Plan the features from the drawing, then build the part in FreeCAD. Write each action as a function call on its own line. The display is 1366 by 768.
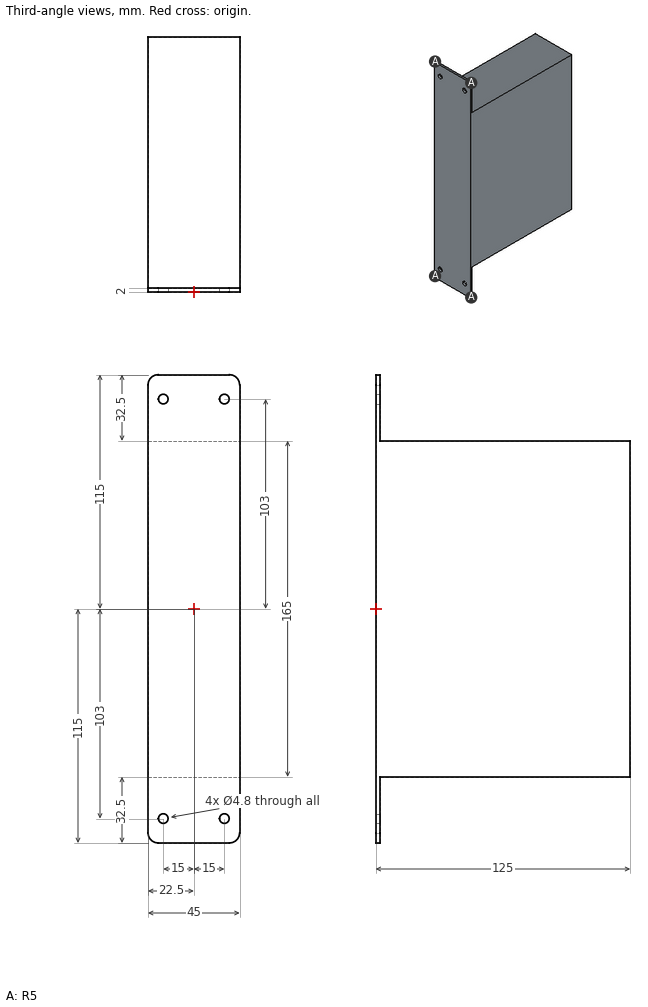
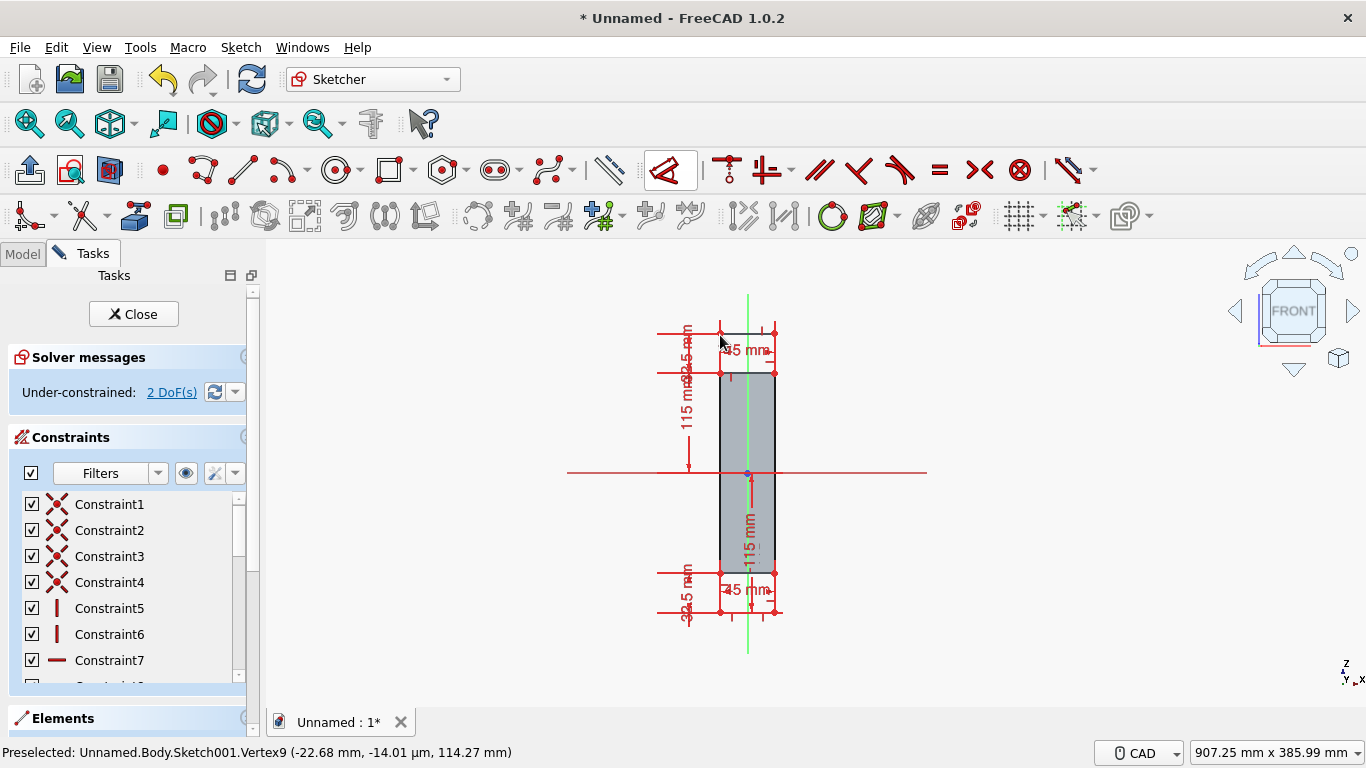
scroll(720, 573, up, 2)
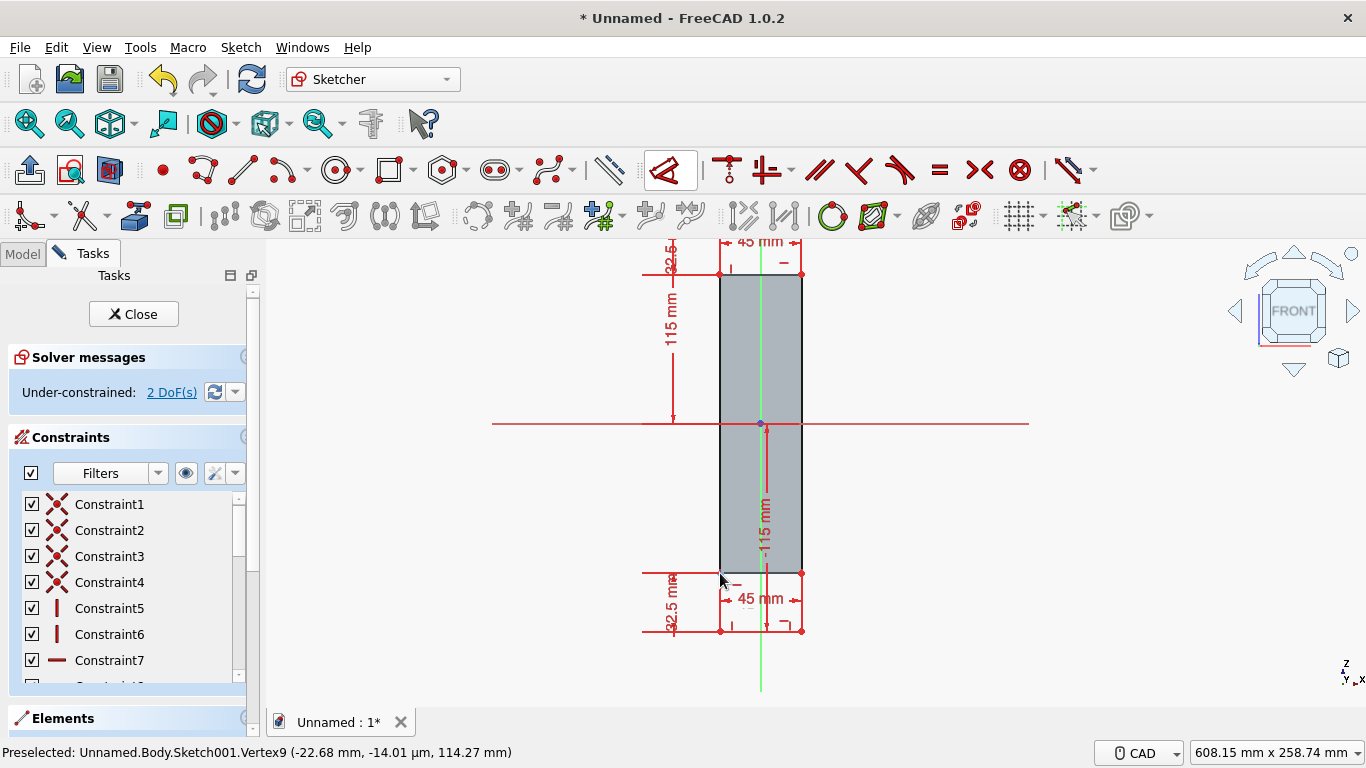
click(720, 573)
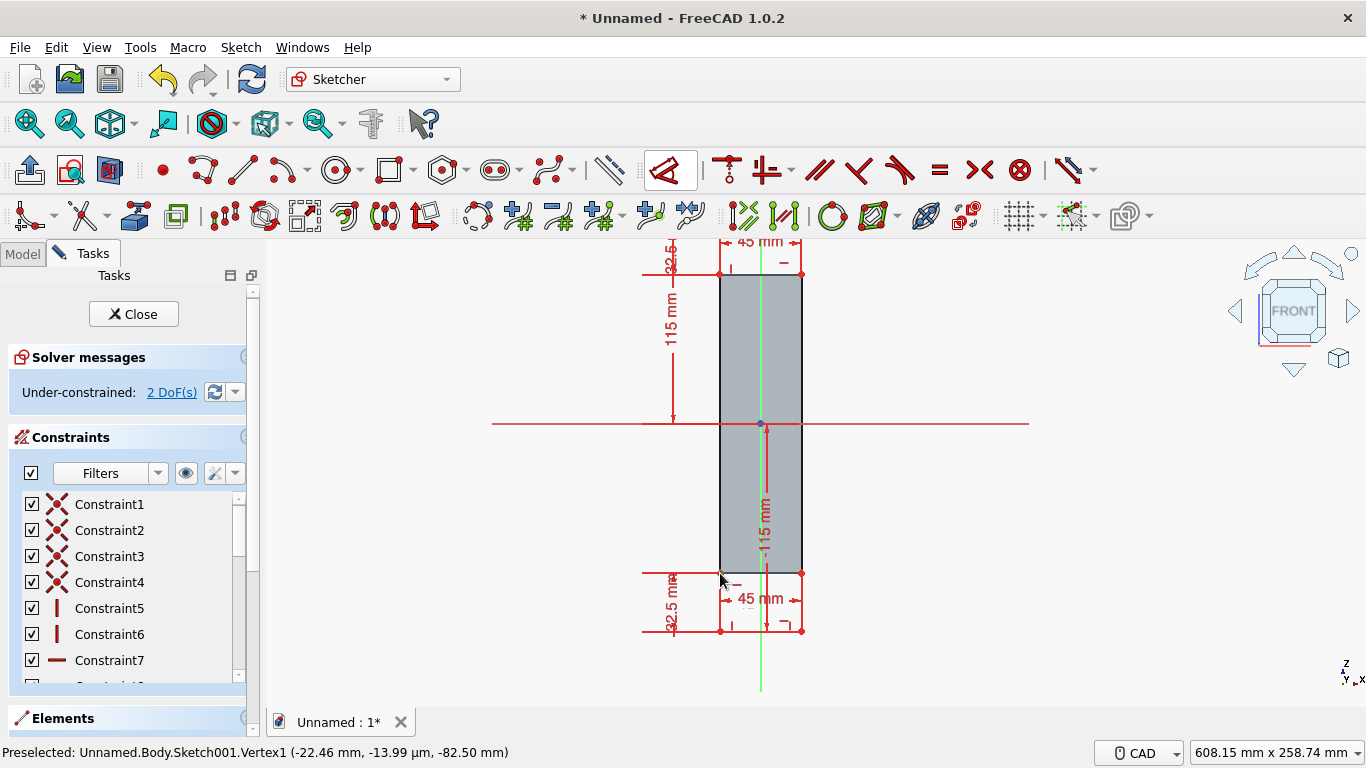
key(l)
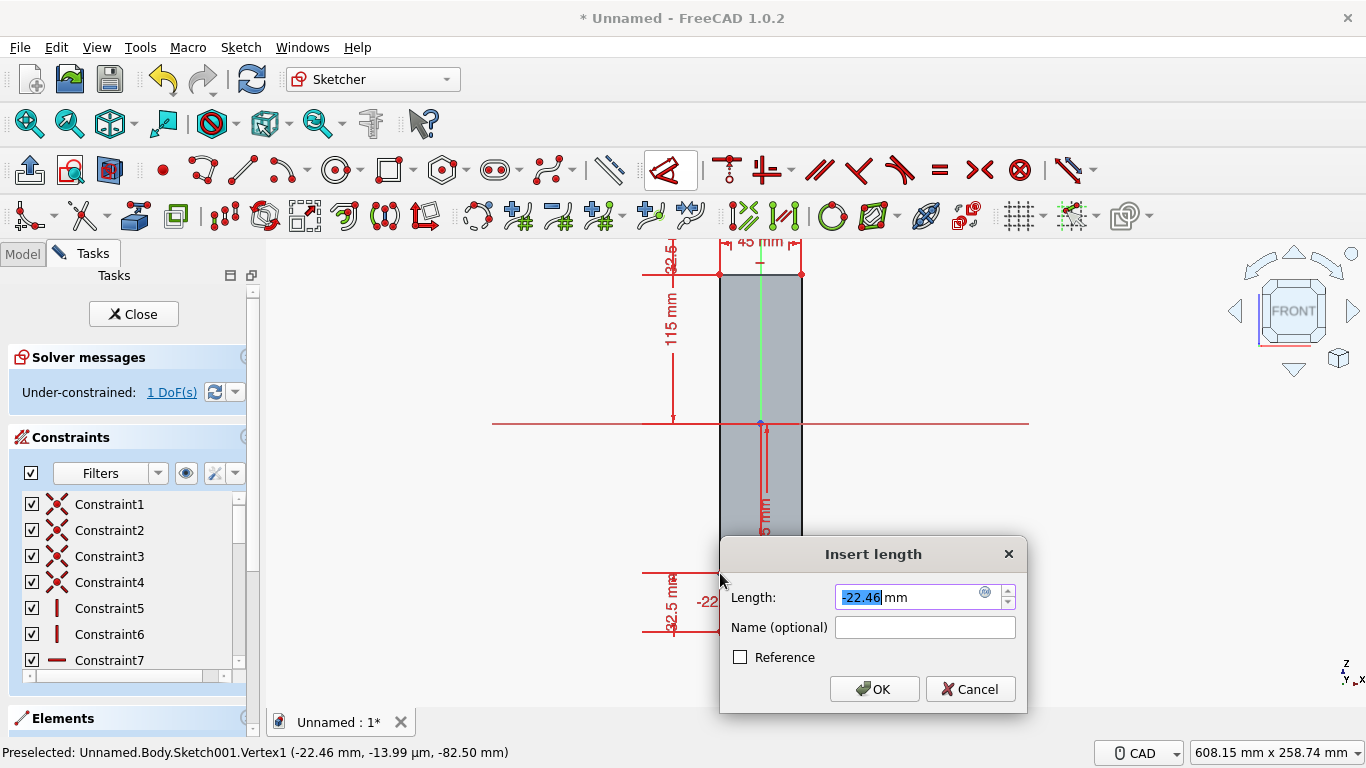
text(-22.5)
key(Return)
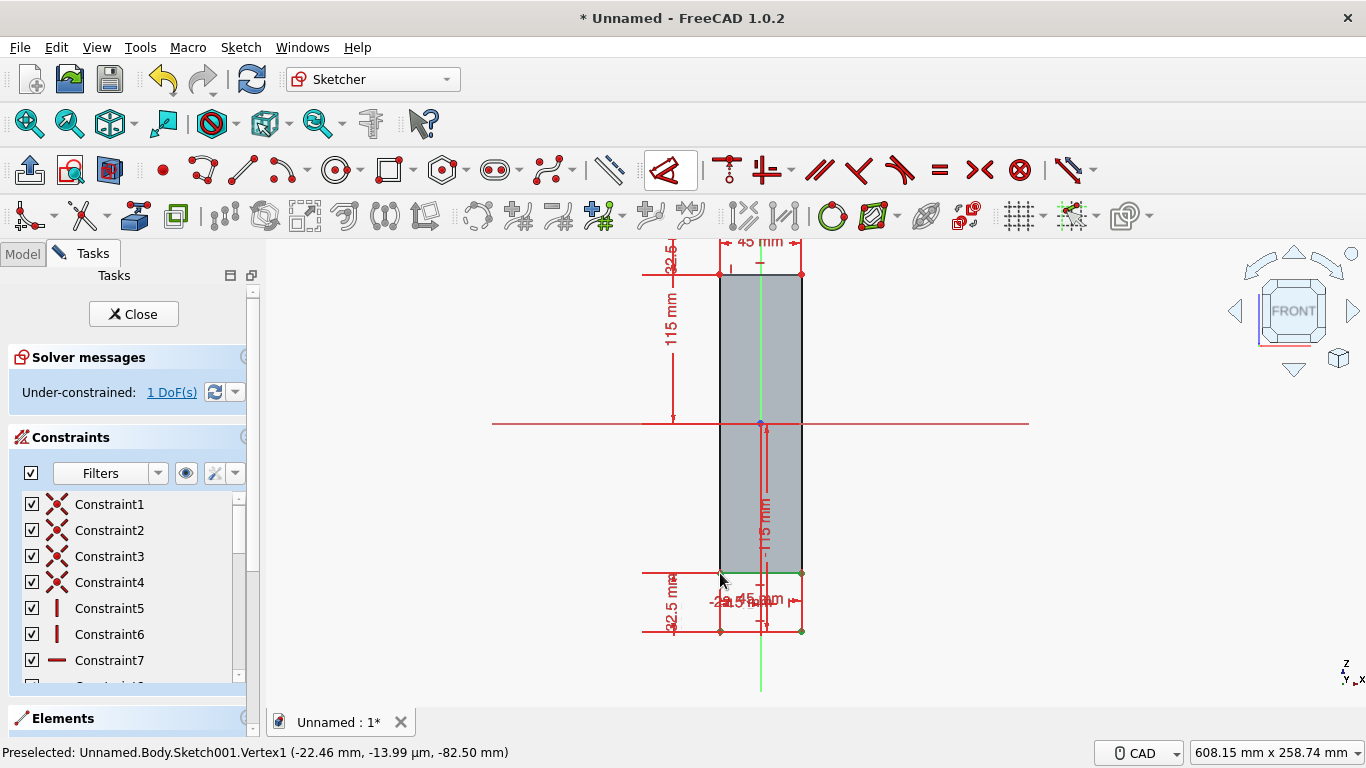
scroll(720, 573, down, 2)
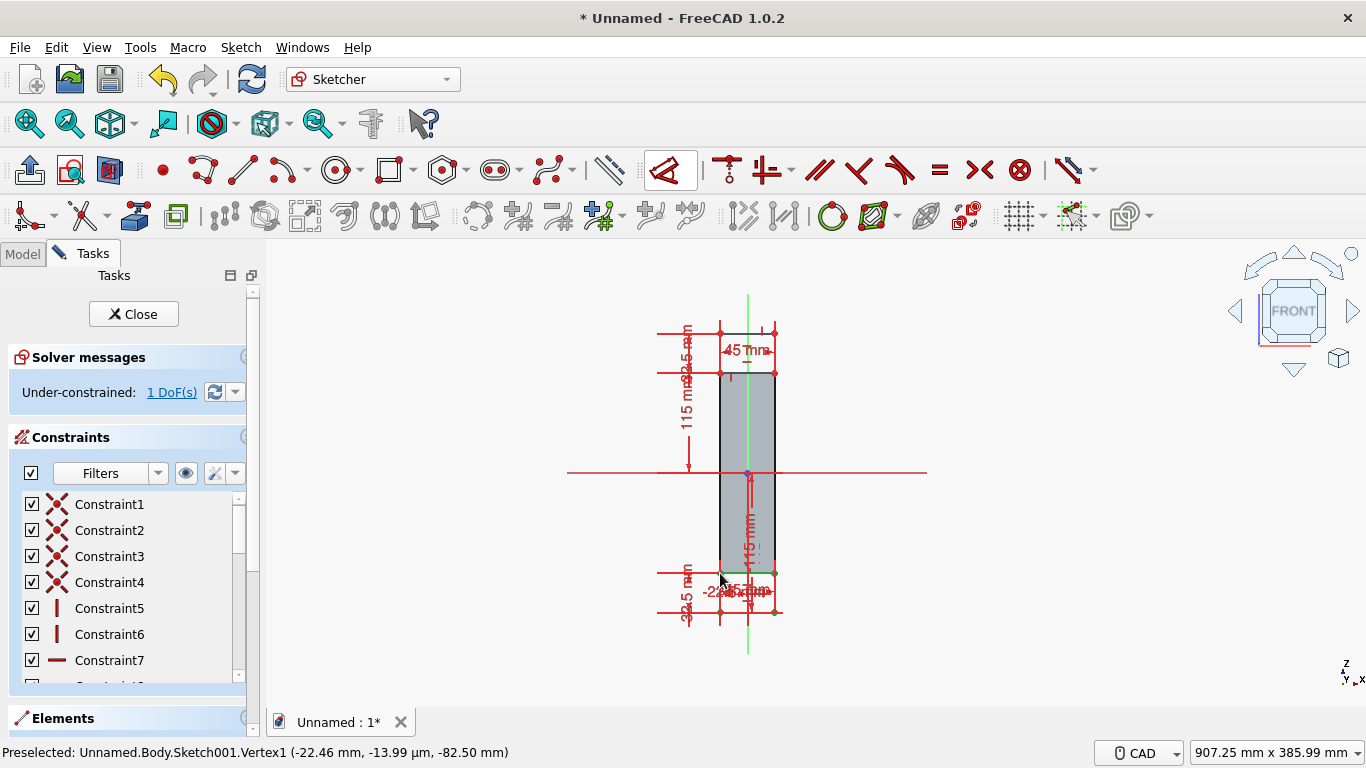
scroll(720, 334, up, 2)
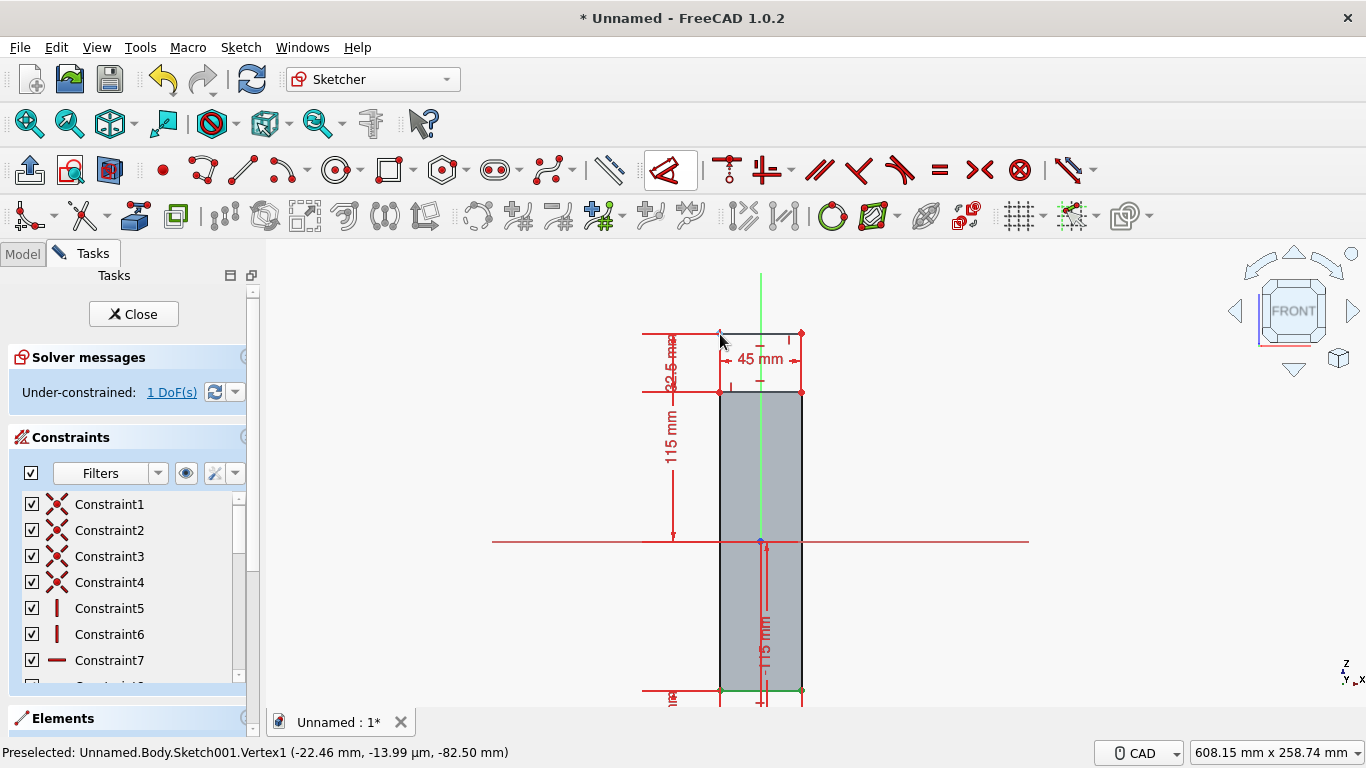
click(720, 334)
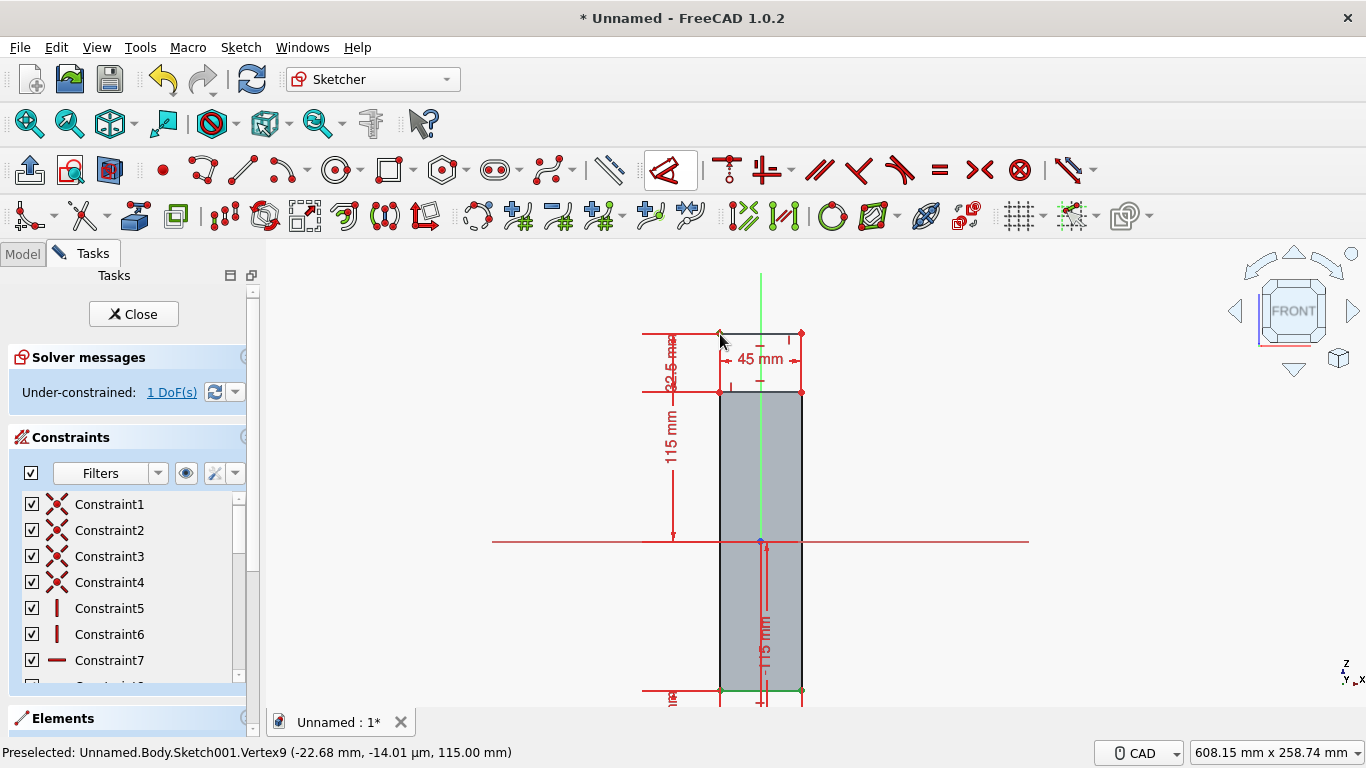
click(692, 170)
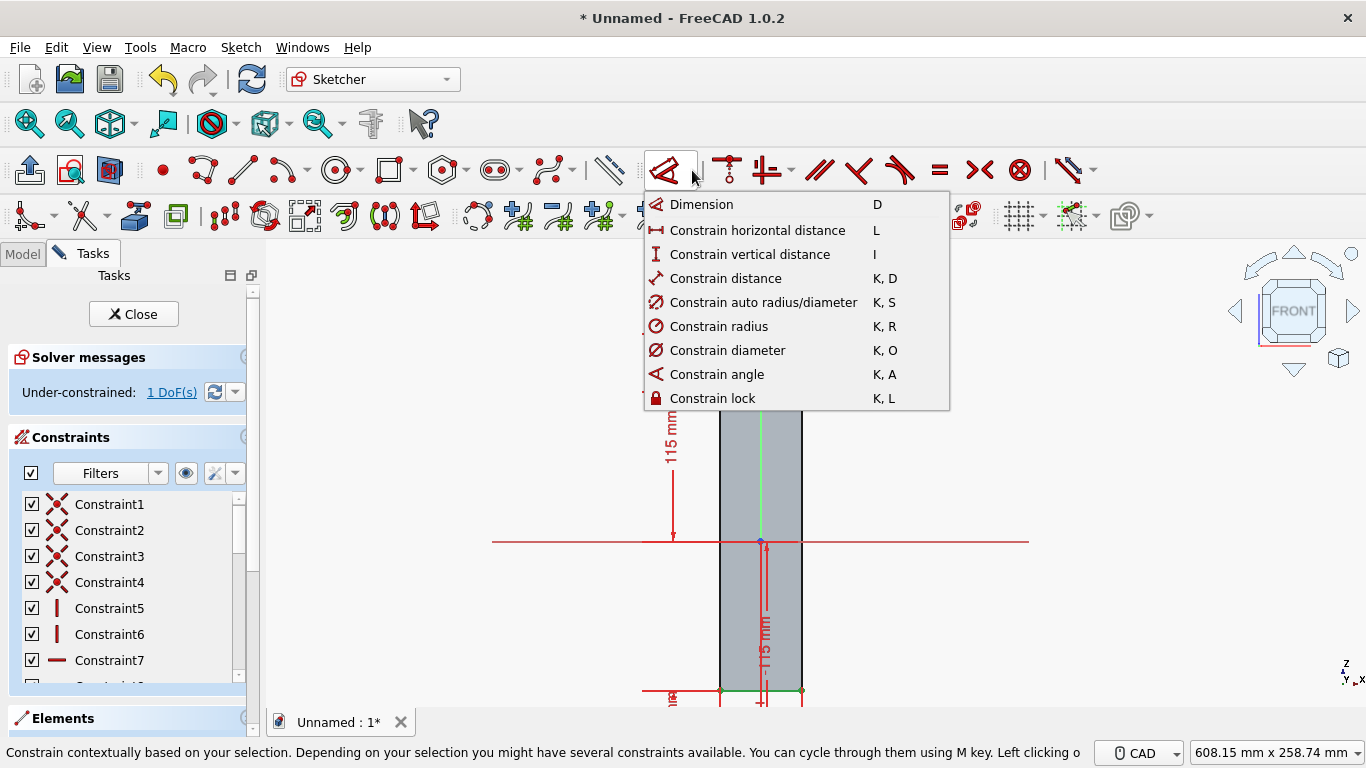
click(797, 230)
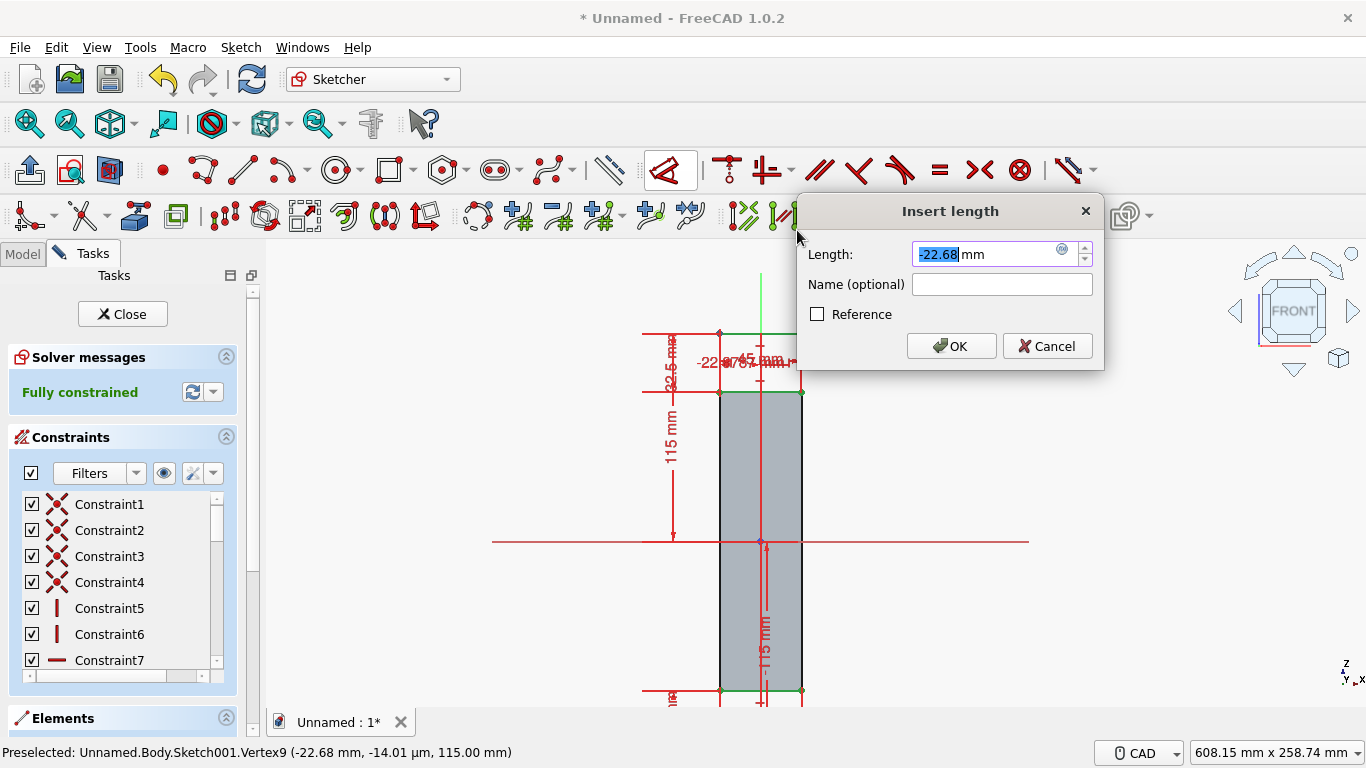
text(-22.5)
key(Return)